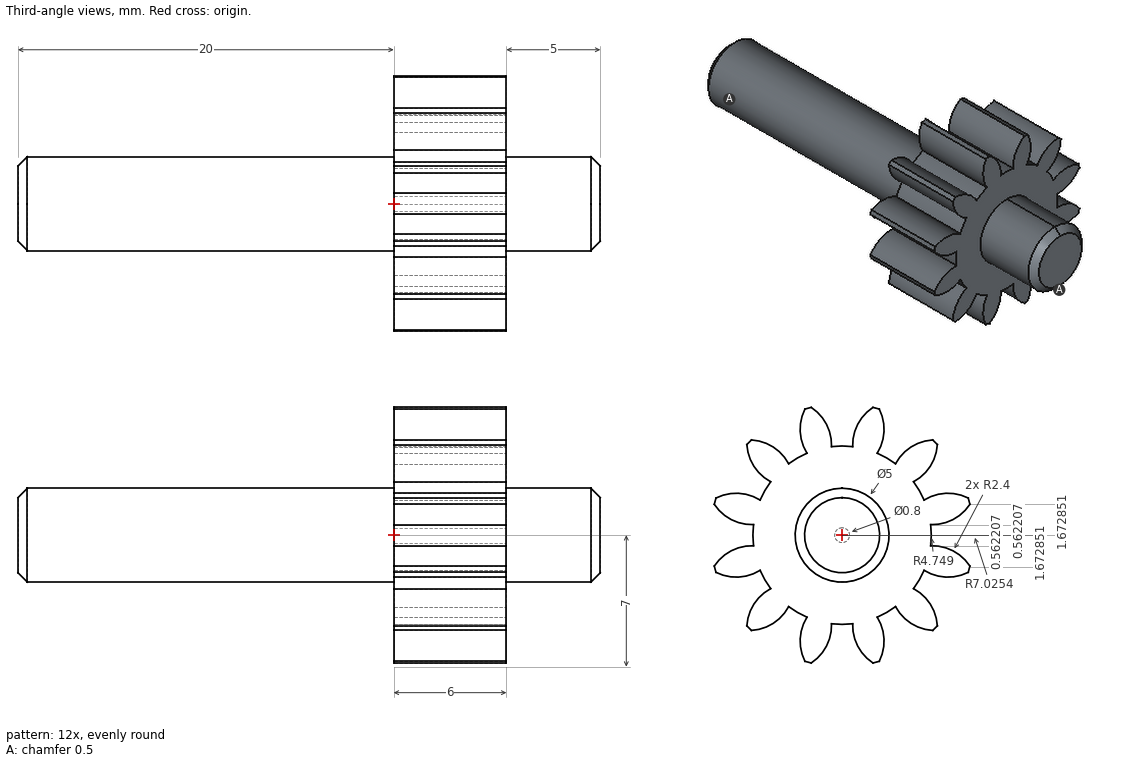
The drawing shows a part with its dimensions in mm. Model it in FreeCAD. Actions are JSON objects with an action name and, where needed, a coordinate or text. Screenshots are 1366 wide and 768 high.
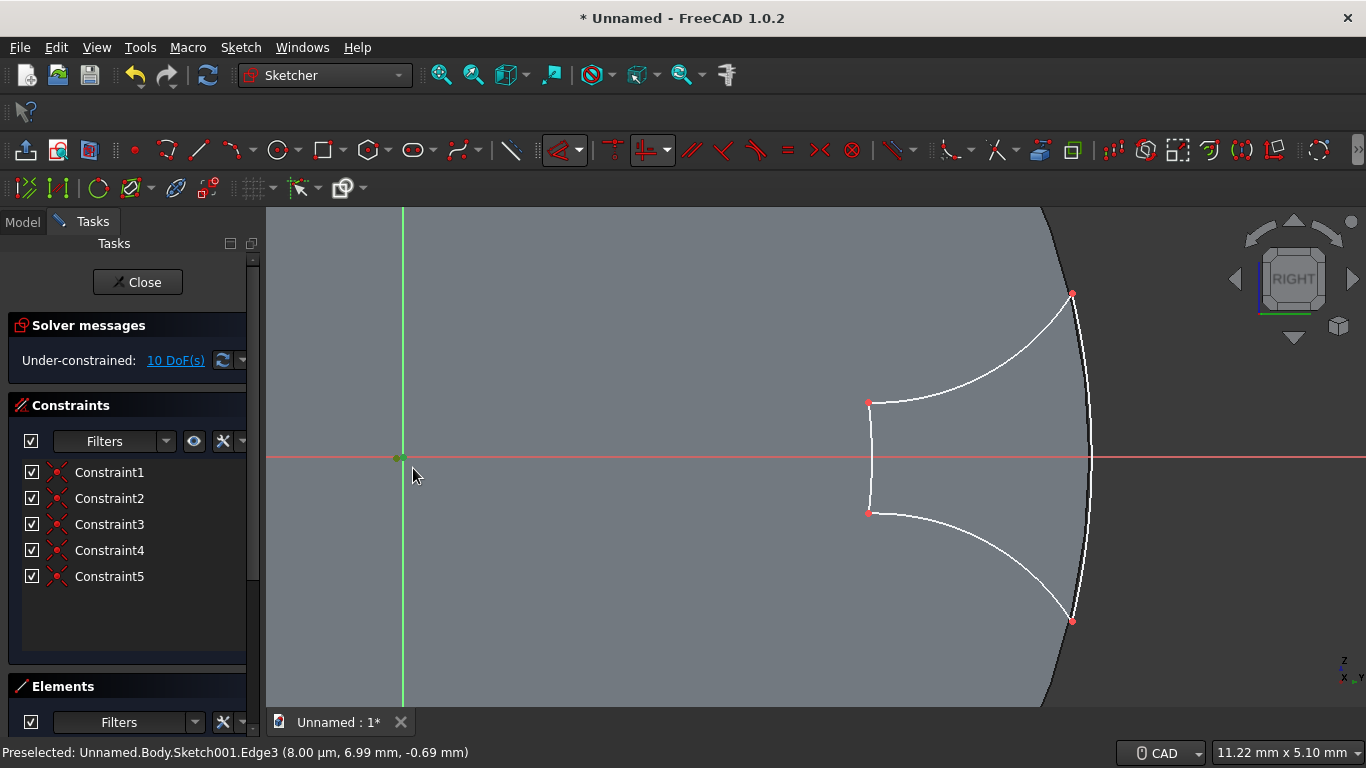
{"action": "left_click", "coordinate": [614, 150]}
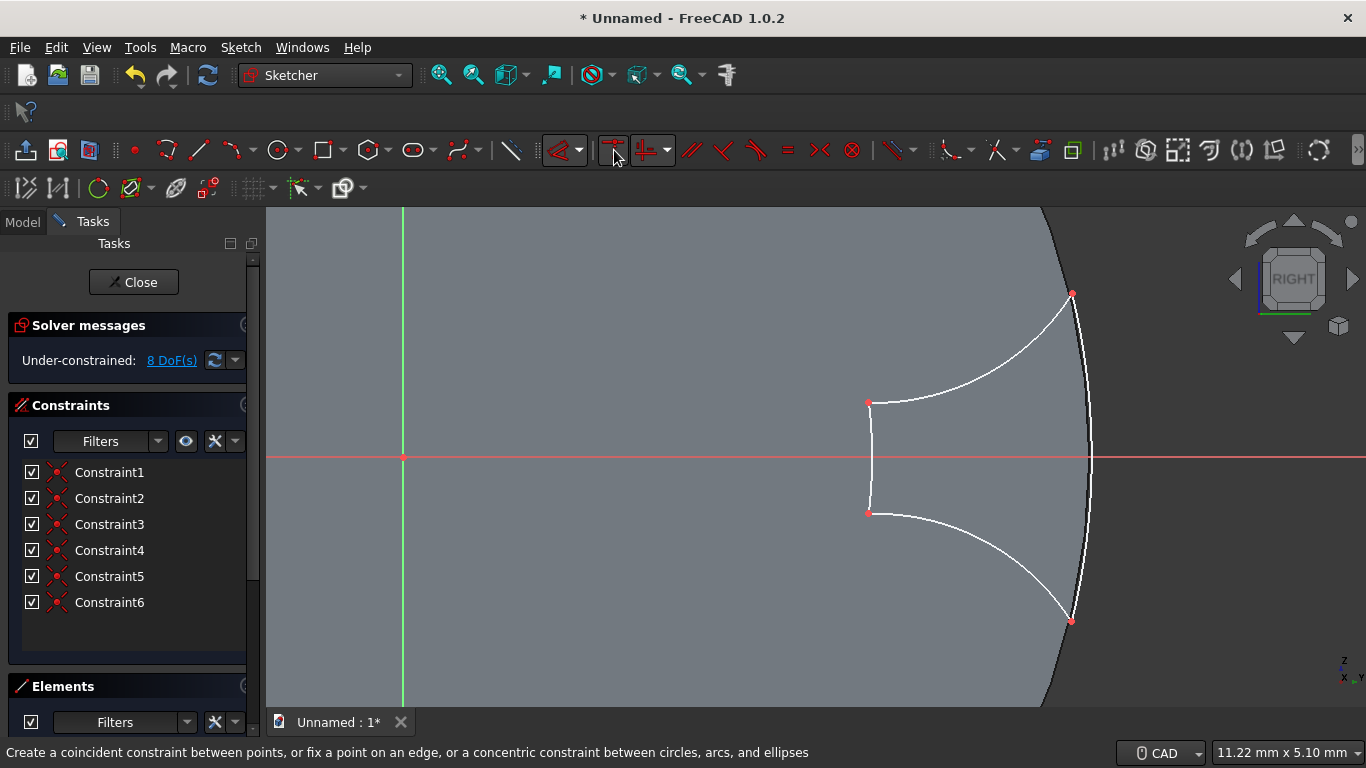
{"action": "left_click", "coordinate": [1024, 568]}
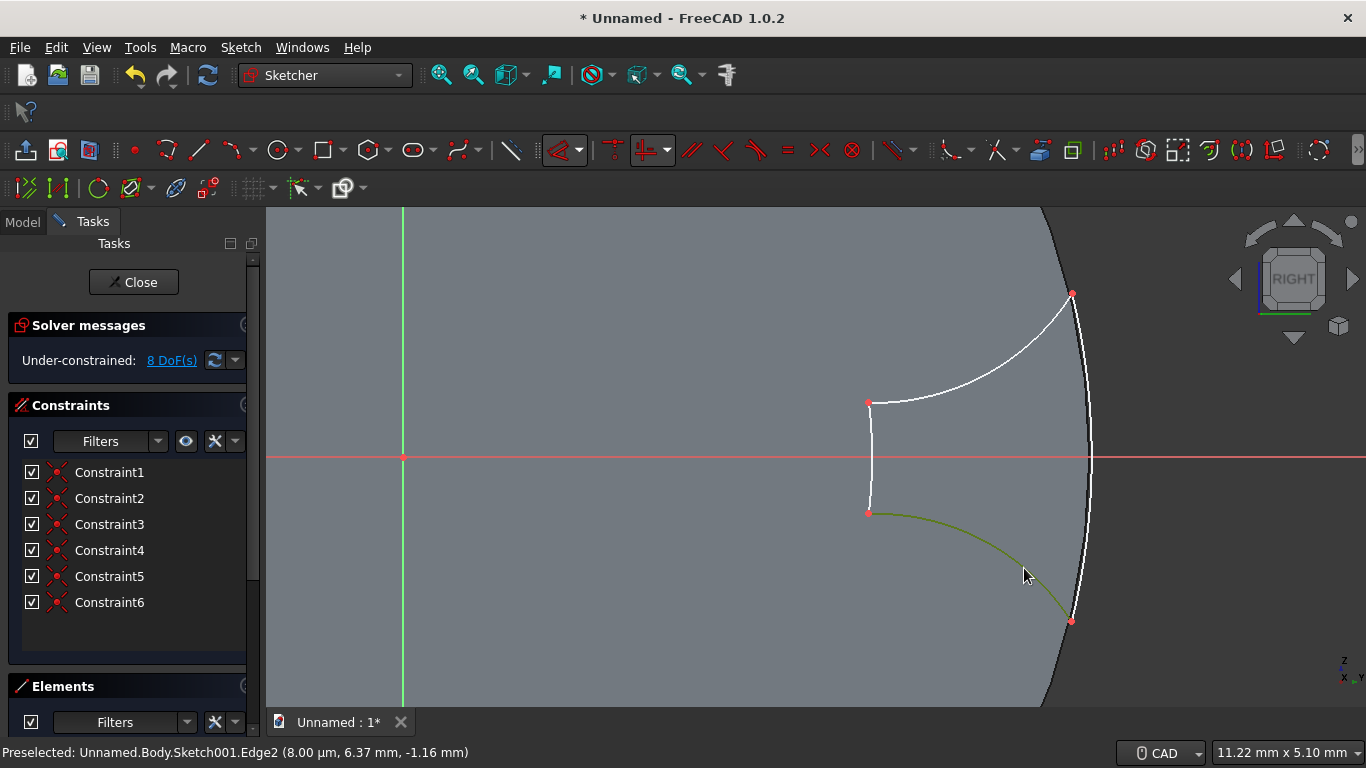
{"action": "left_click", "coordinate": [940, 393]}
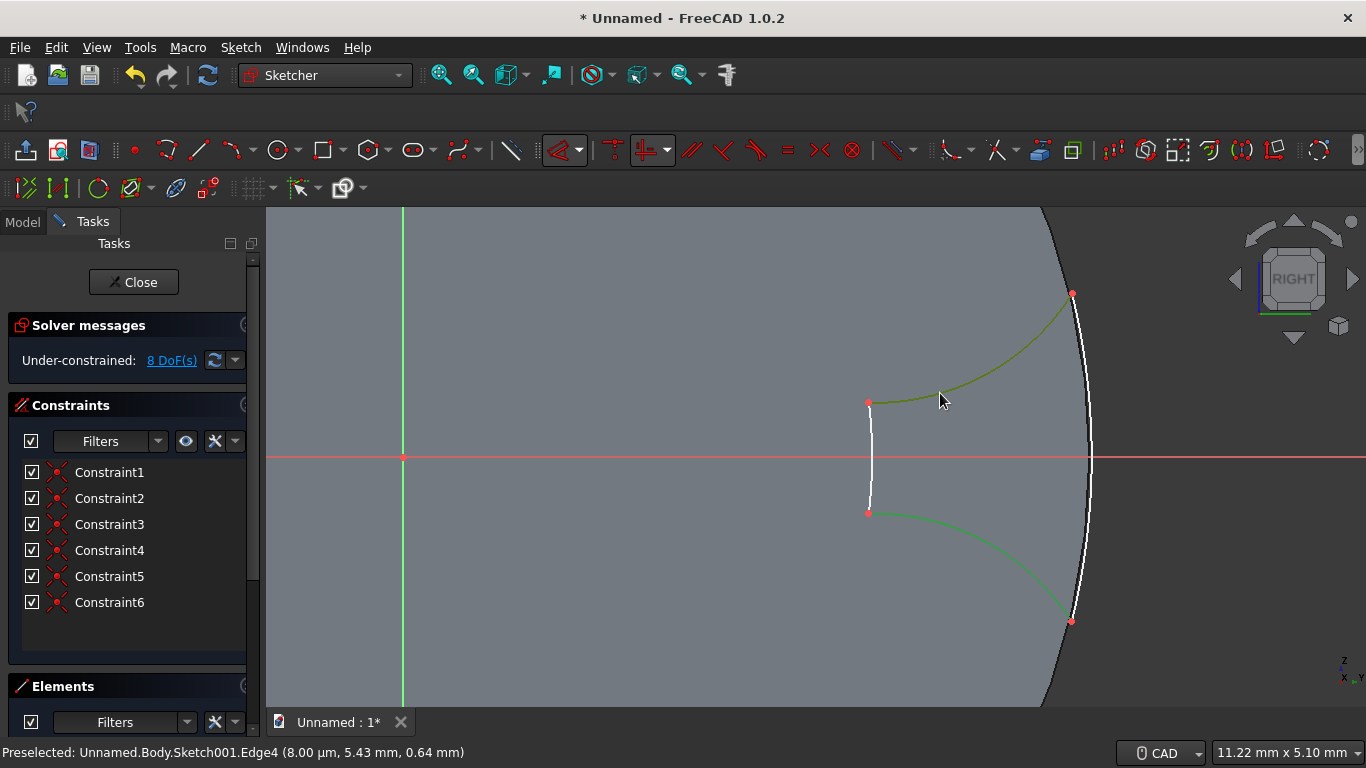
{"action": "left_click", "coordinate": [788, 150]}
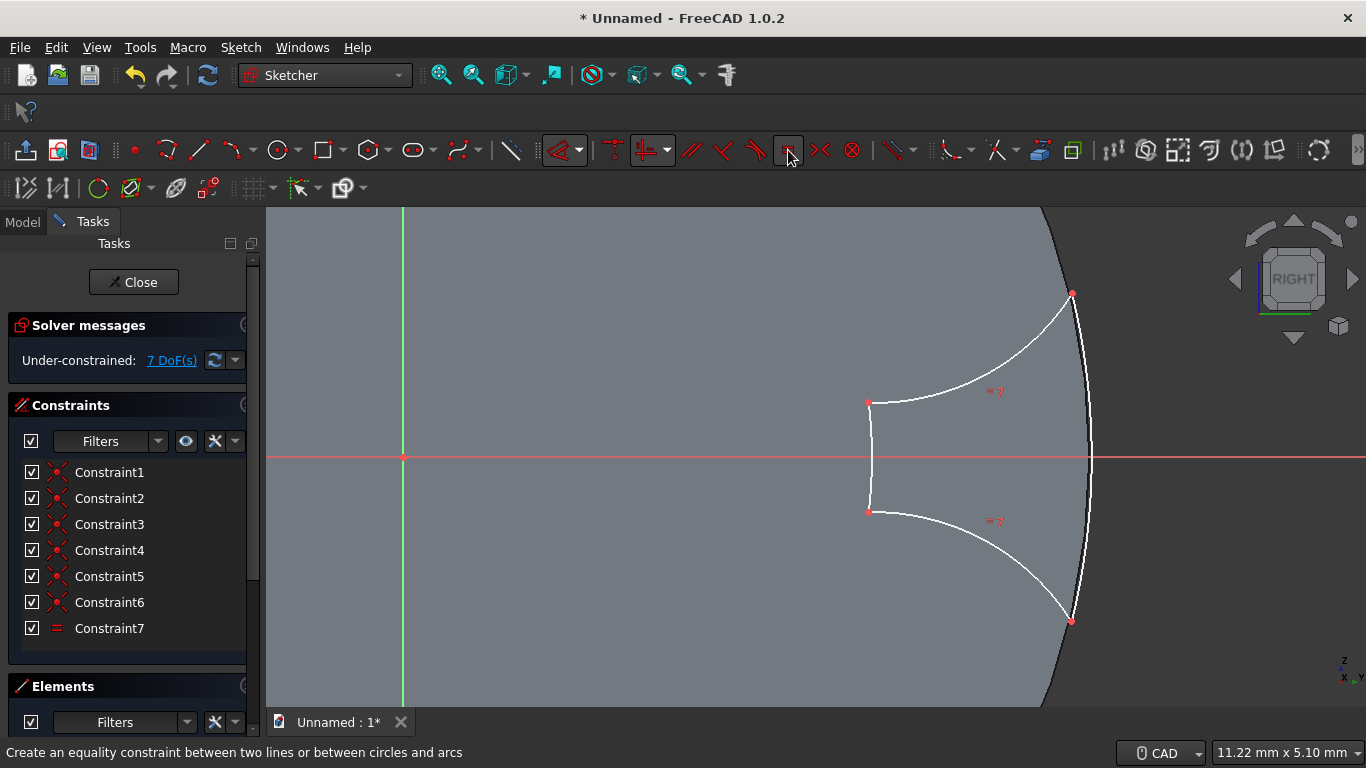
{"action": "left_click", "coordinate": [871, 479]}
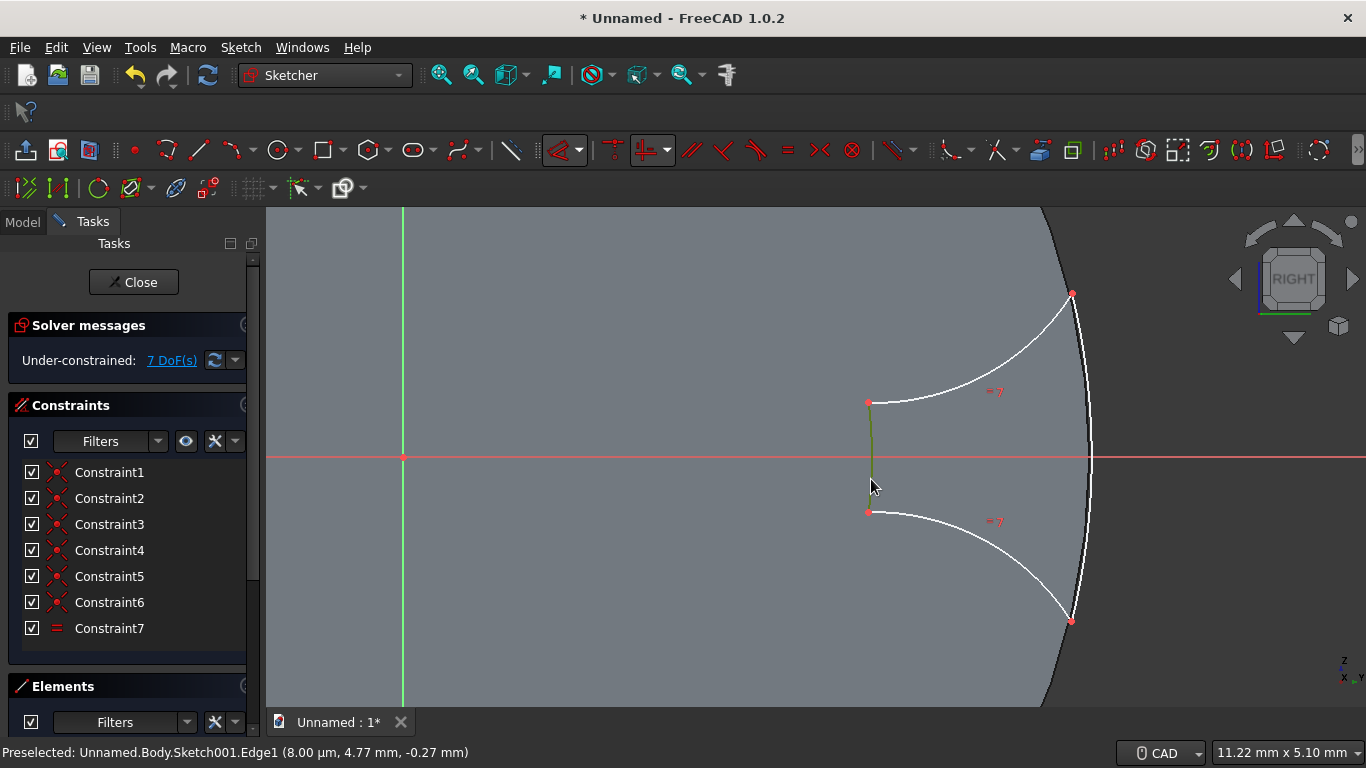
{"action": "key", "text": "k r"}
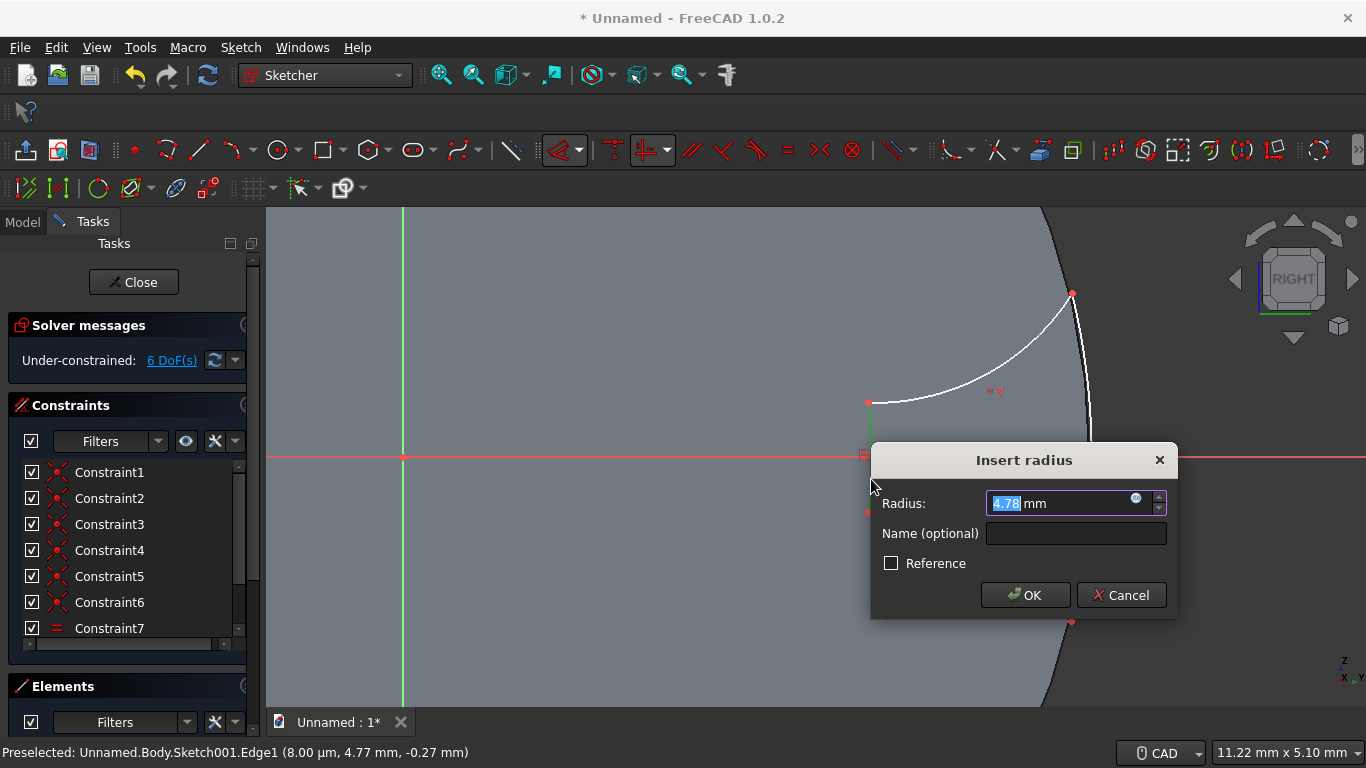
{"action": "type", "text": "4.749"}
{"action": "key", "text": "Return"}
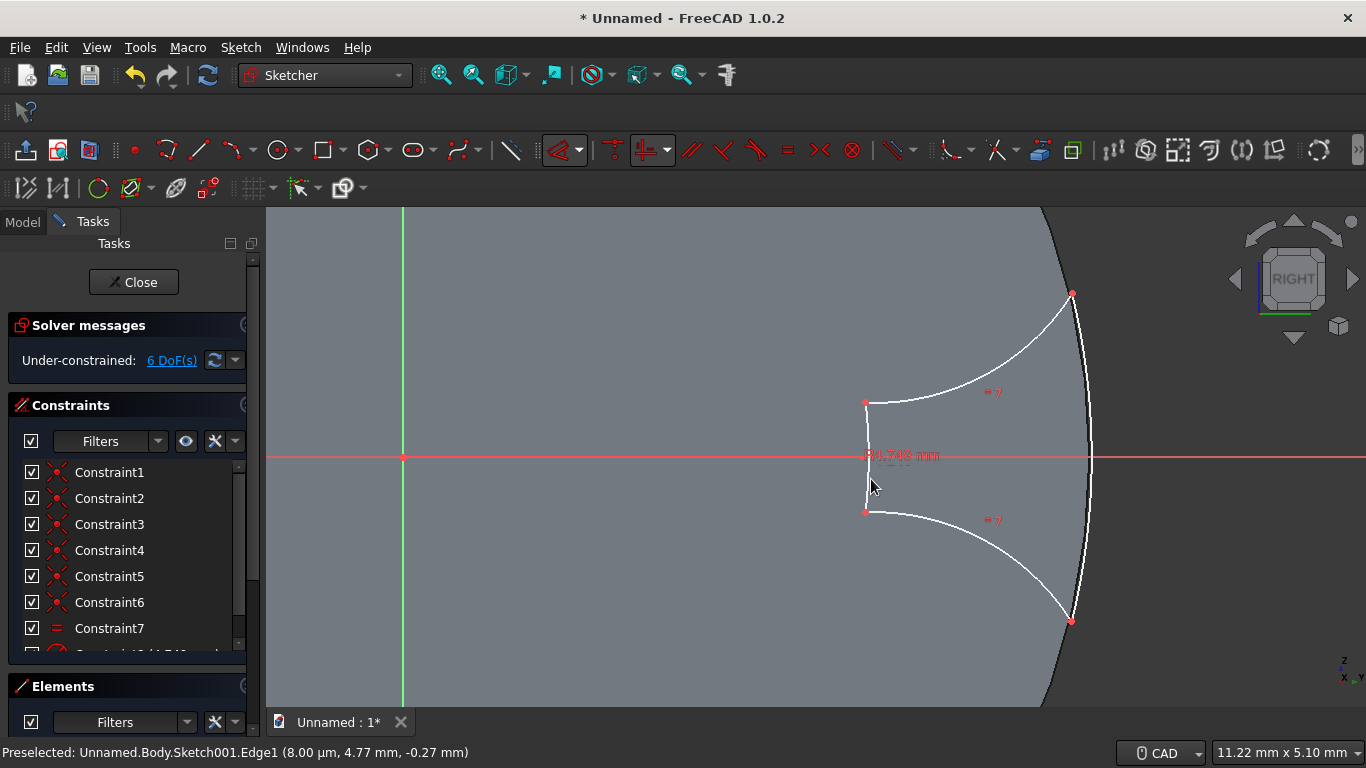
{"action": "left_click", "coordinate": [1024, 567]}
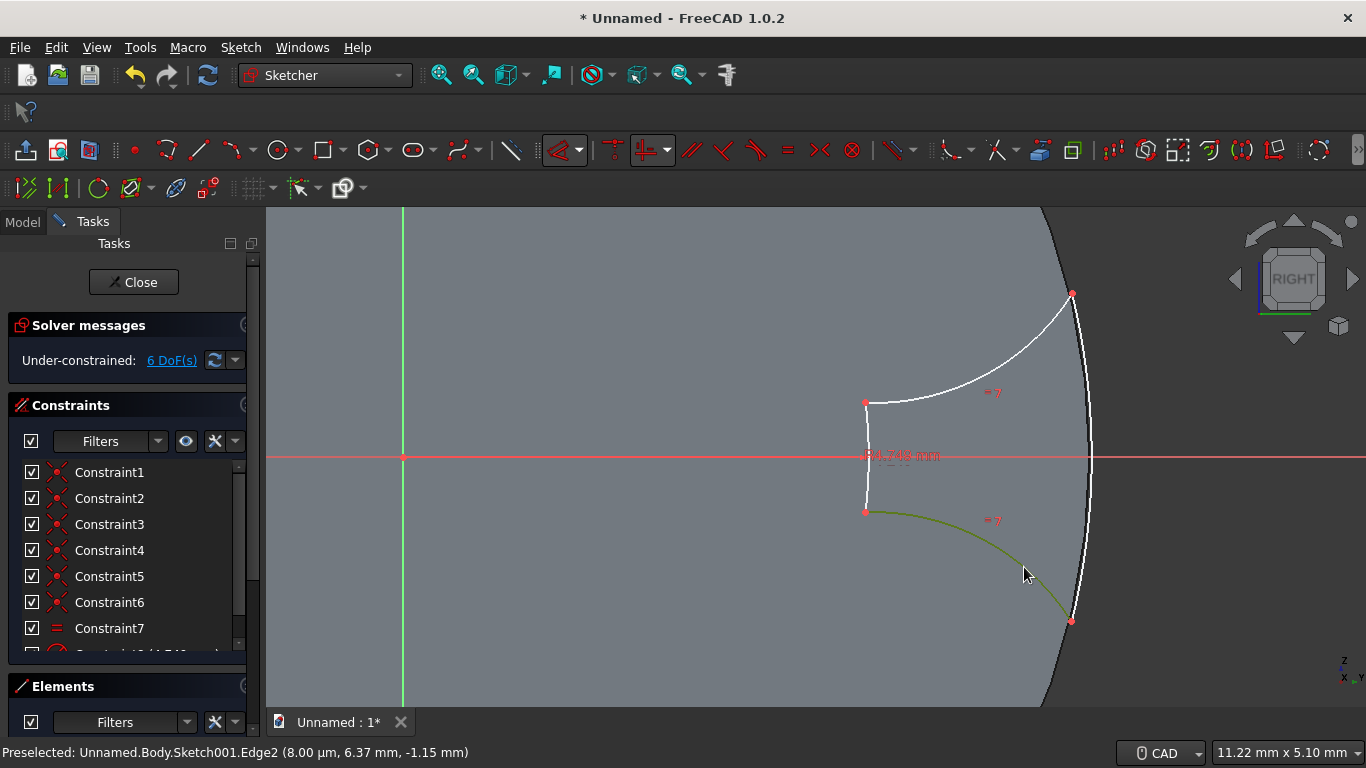
{"action": "key", "text": "k r"}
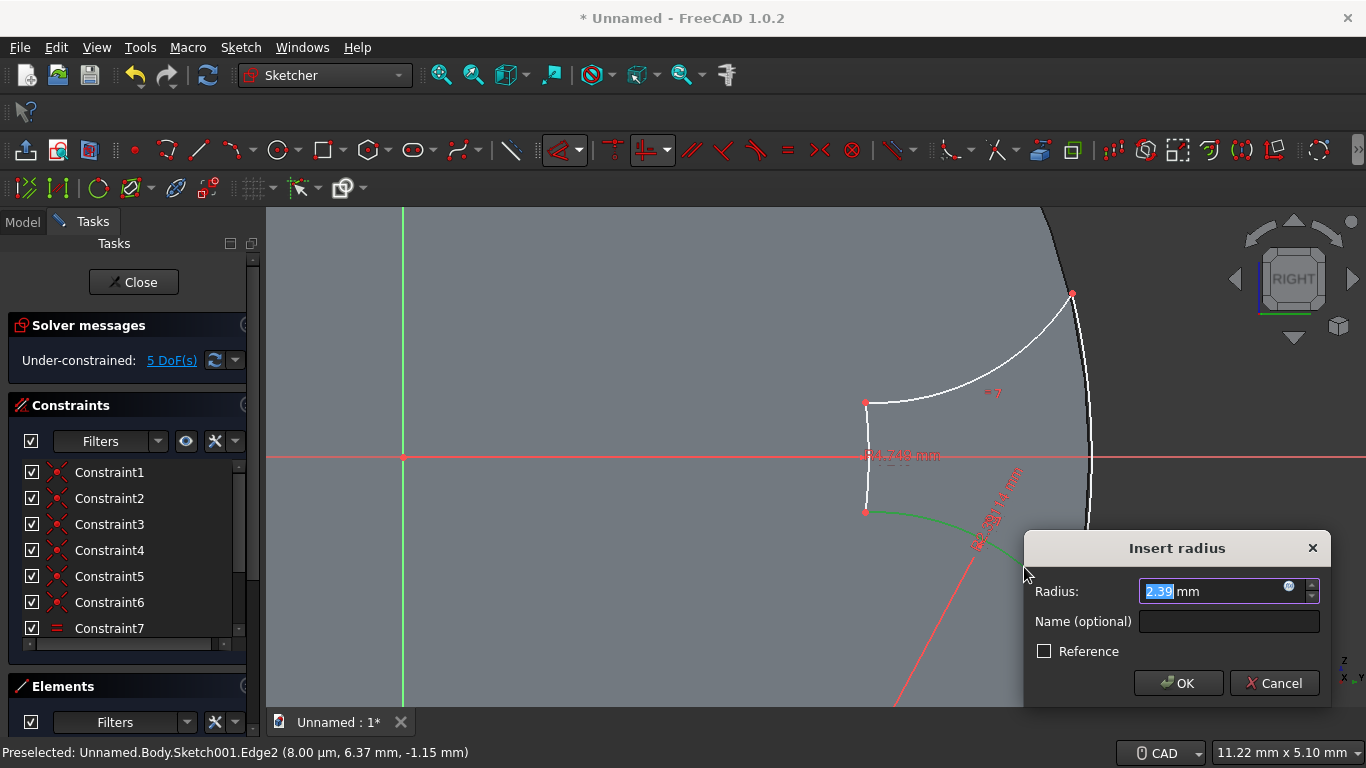
{"action": "type", "text": "2.4"}
{"action": "key", "text": "Return"}